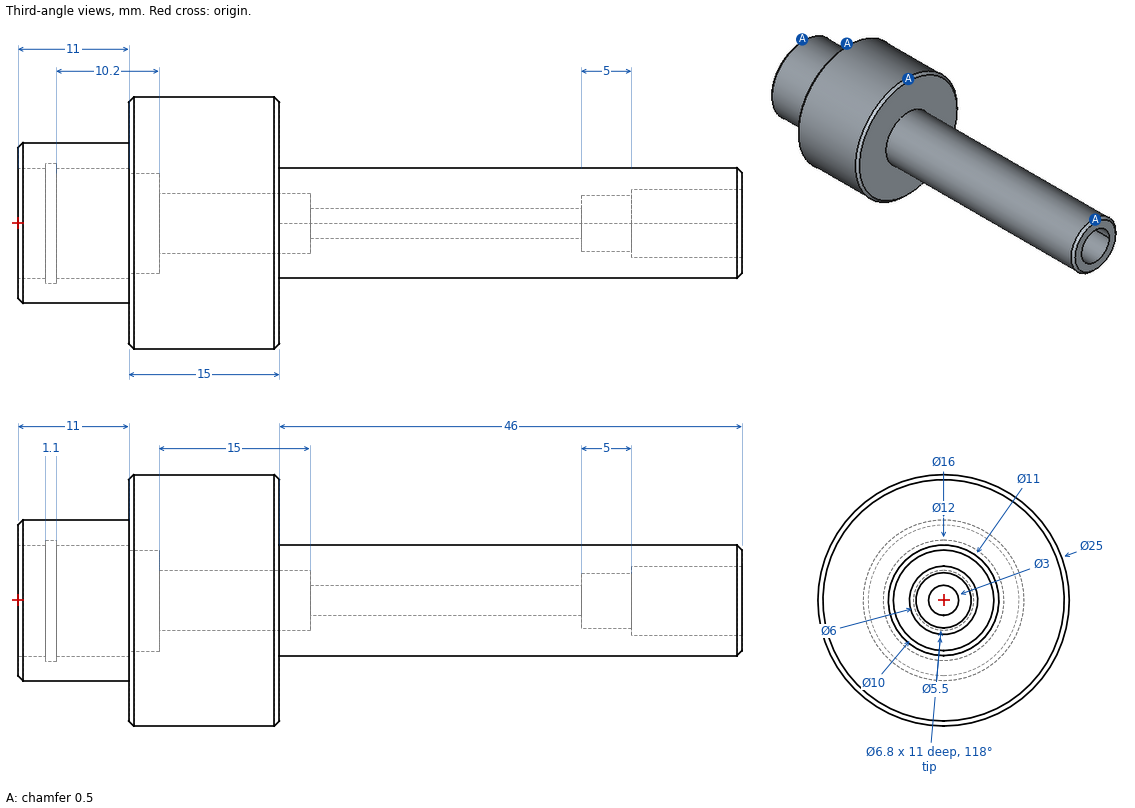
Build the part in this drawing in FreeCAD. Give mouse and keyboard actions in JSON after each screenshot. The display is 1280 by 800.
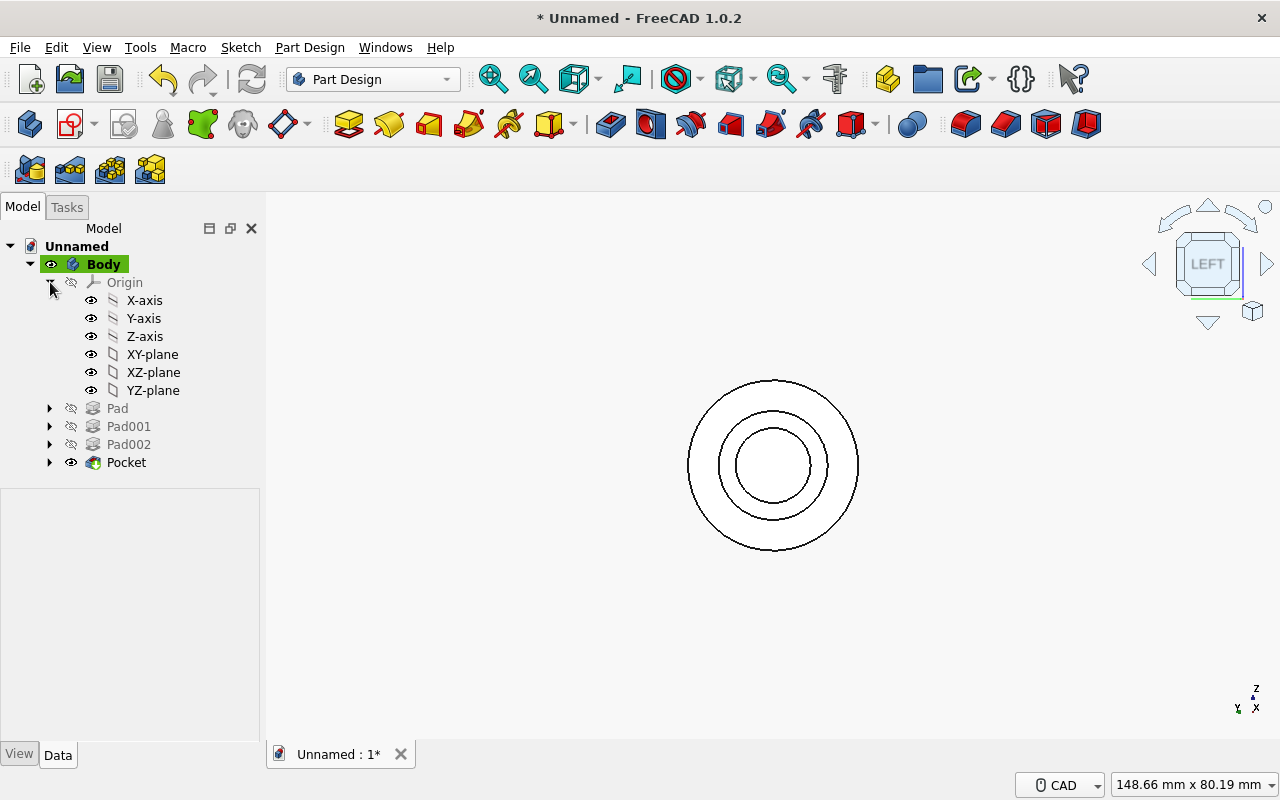
{"action": "left_click", "coordinate": [136, 390]}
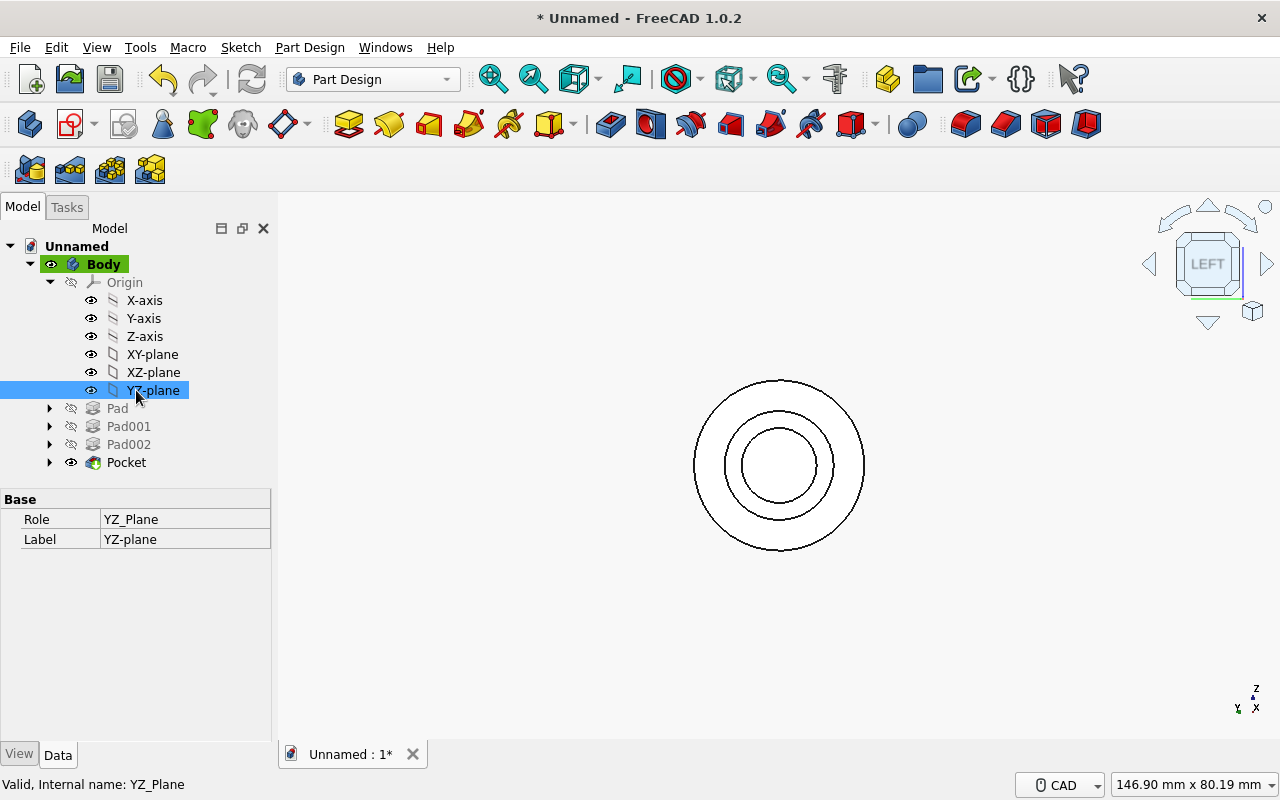
{"action": "left_click", "coordinate": [284, 124]}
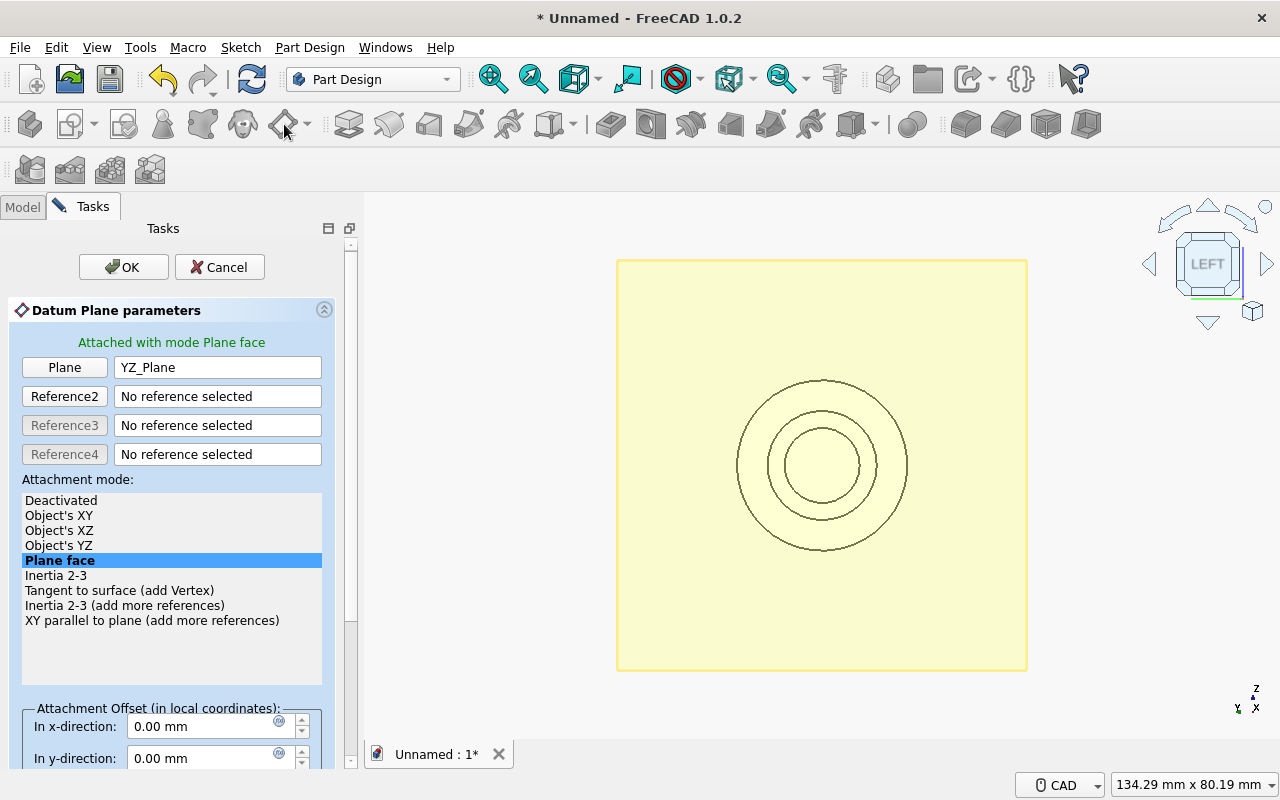
{"action": "scroll", "coordinate": [351, 503], "scroll_direction": "down", "scroll_amount": 2}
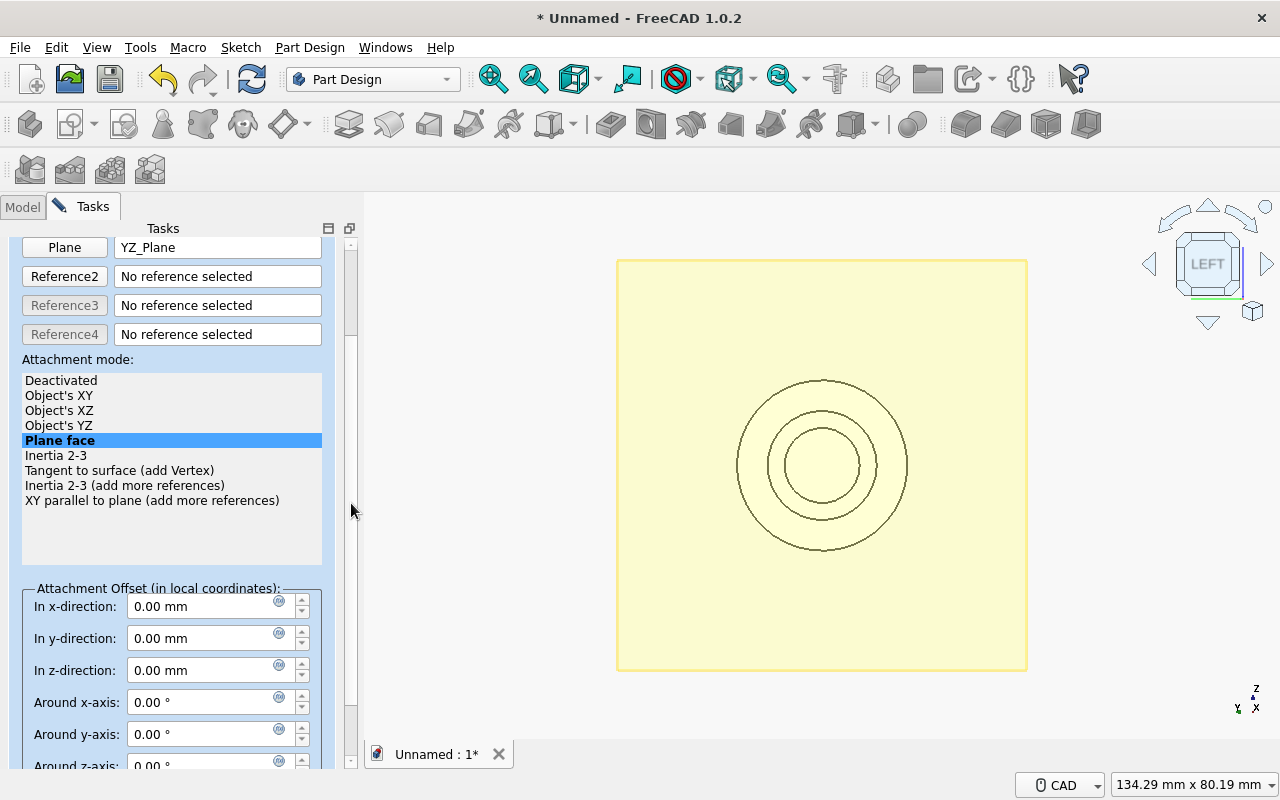
{"action": "triple_click", "coordinate": [210, 670]}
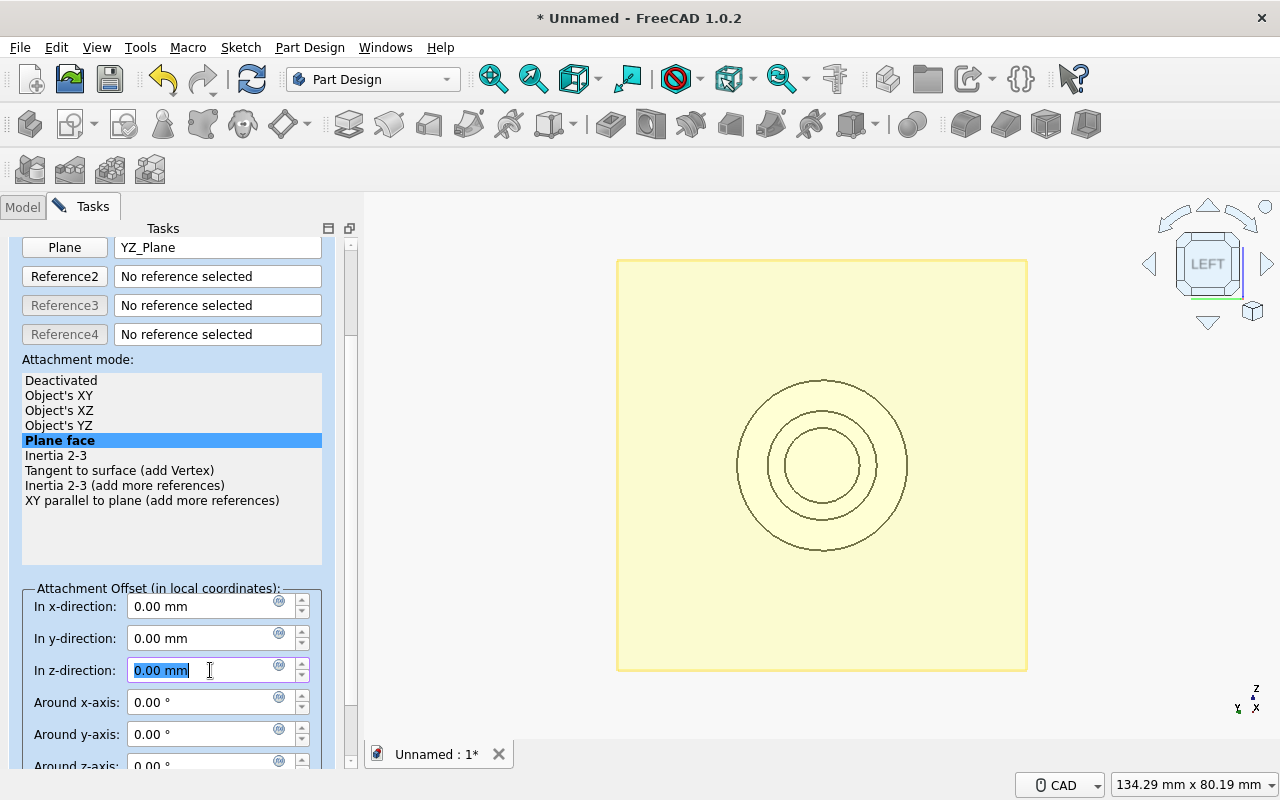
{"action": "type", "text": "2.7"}
{"action": "key", "text": "Tab"}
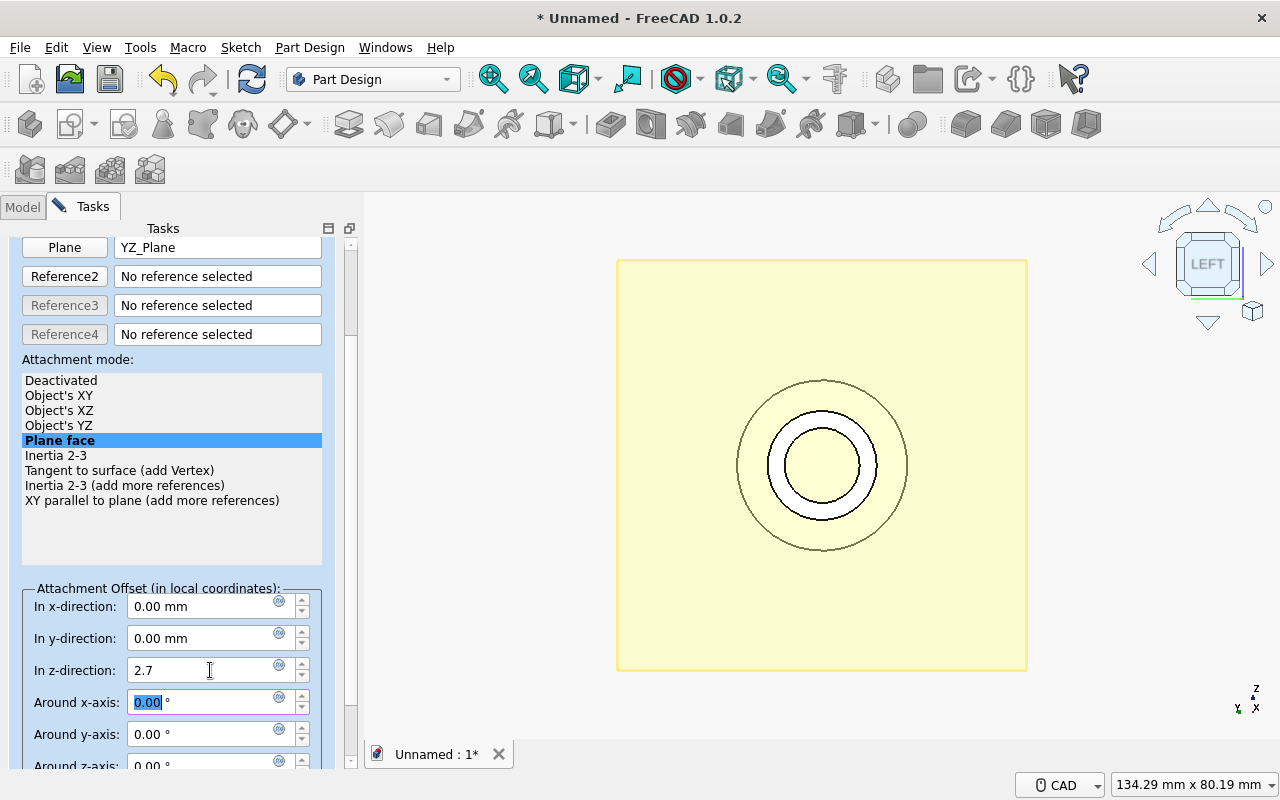
{"action": "scroll", "coordinate": [351, 503], "scroll_direction": "up", "scroll_amount": 3}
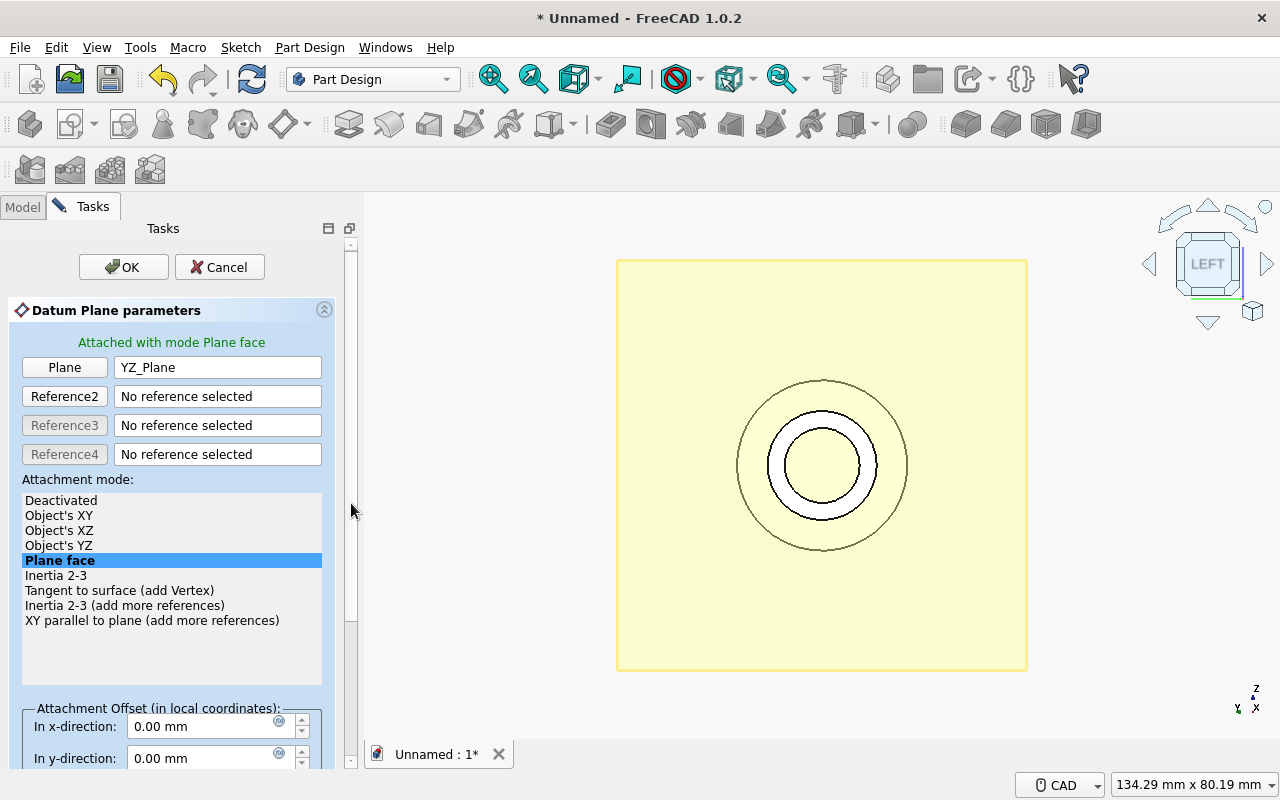
{"action": "left_click", "coordinate": [124, 267]}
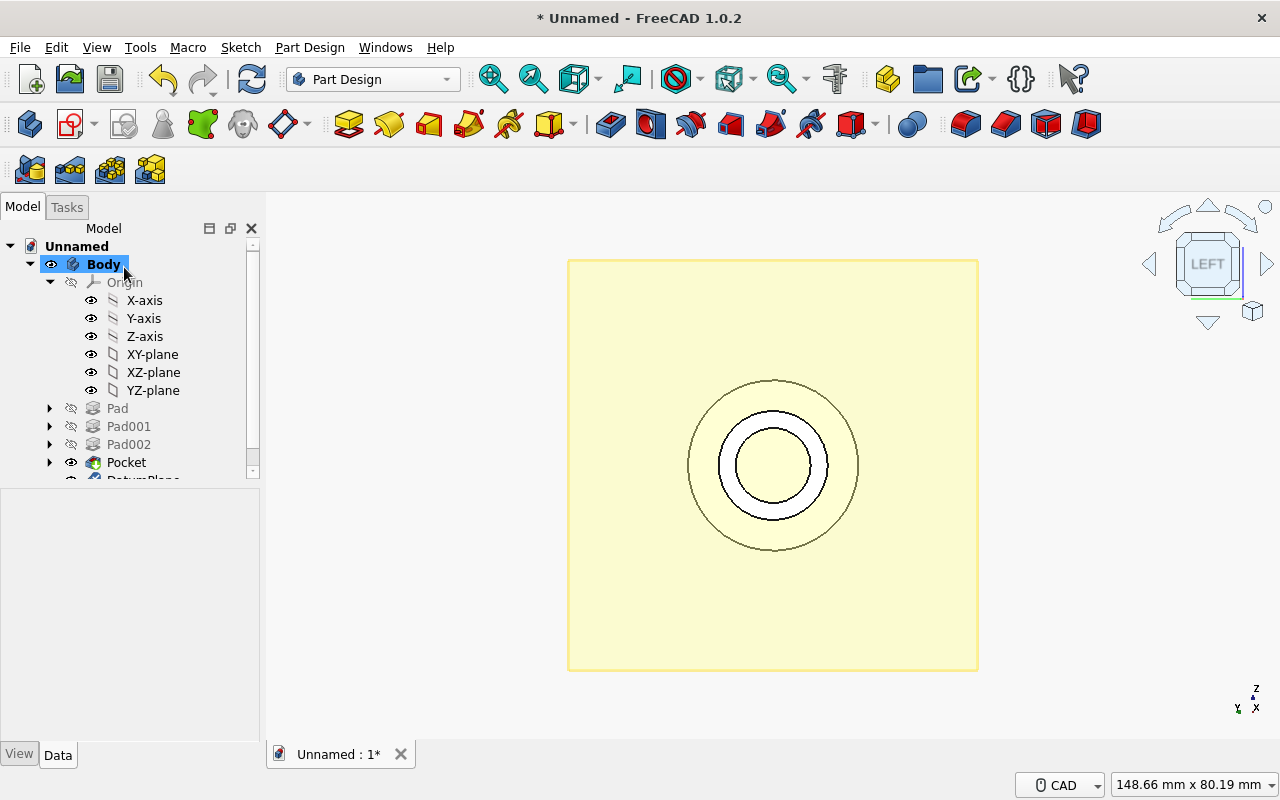
{"action": "scroll", "coordinate": [100, 350], "scroll_direction": "down", "scroll_amount": 3}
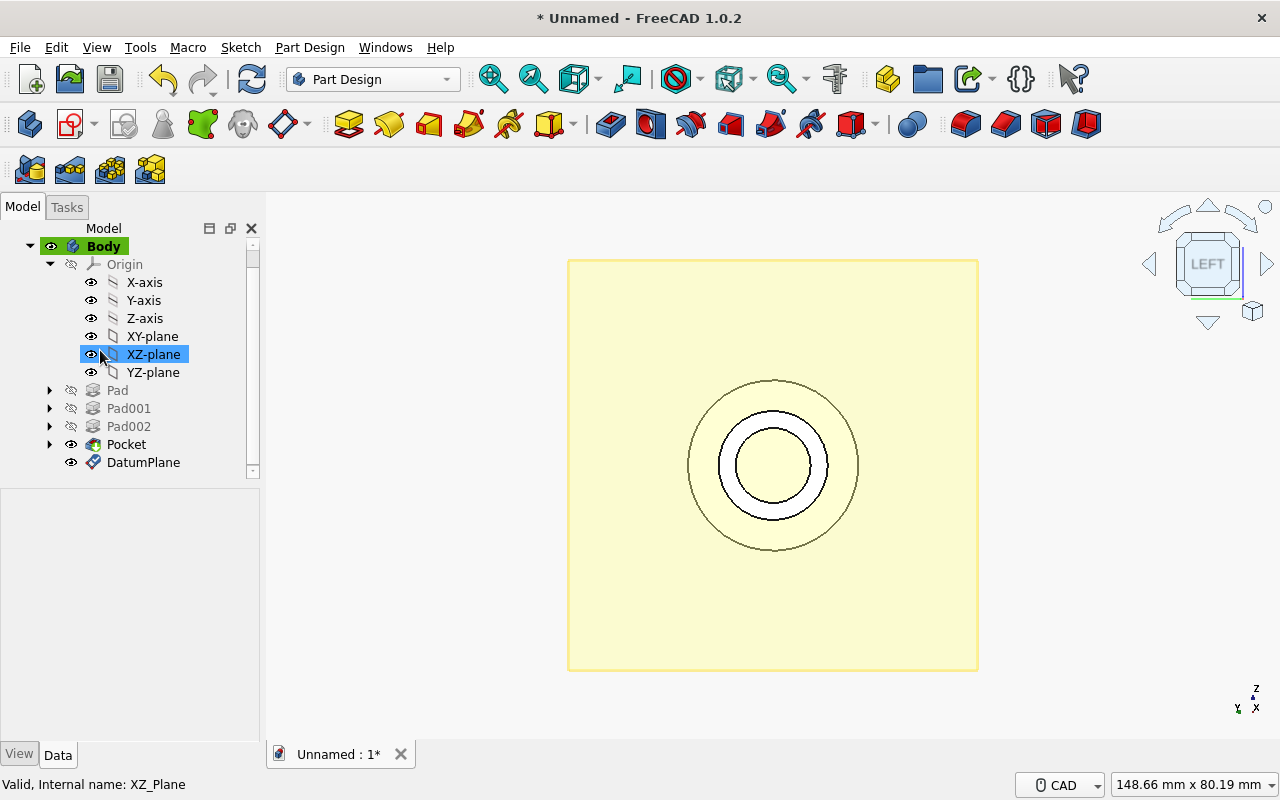
{"action": "left_click", "coordinate": [116, 462]}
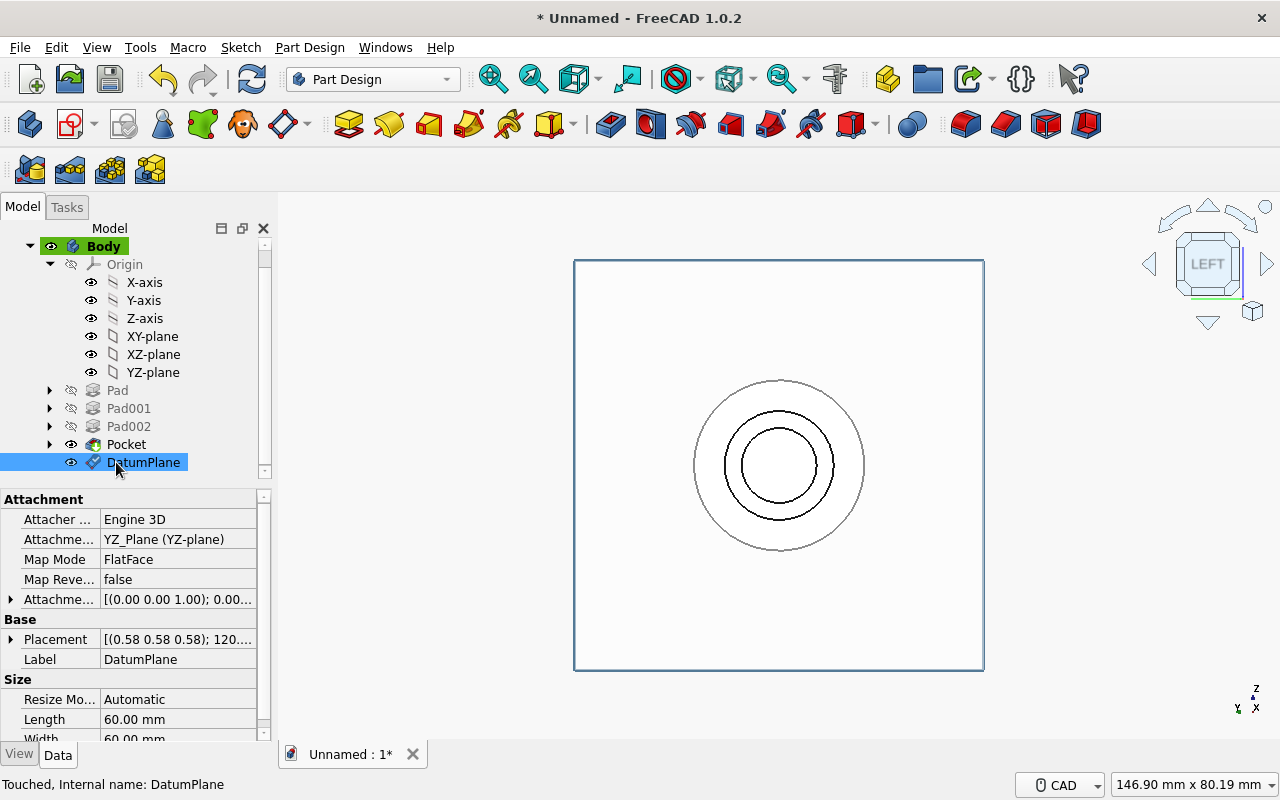
{"action": "left_click", "coordinate": [70, 124]}